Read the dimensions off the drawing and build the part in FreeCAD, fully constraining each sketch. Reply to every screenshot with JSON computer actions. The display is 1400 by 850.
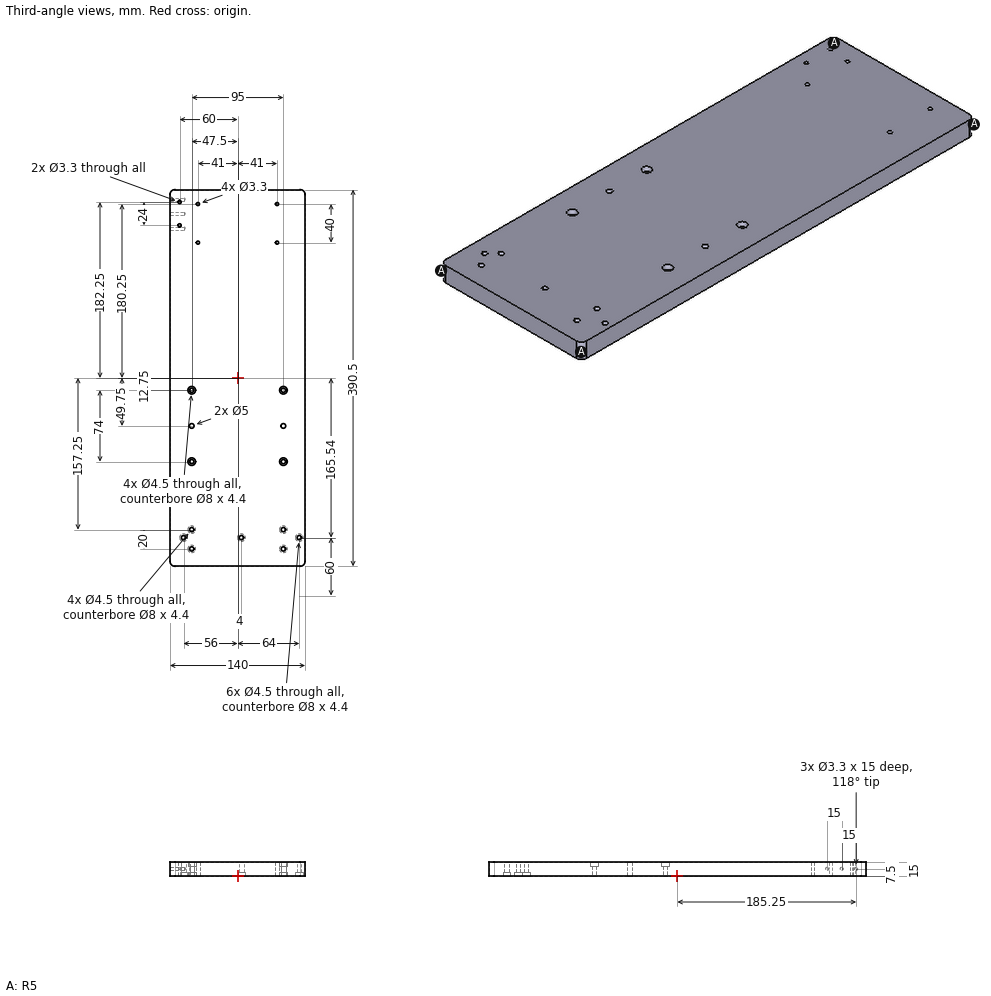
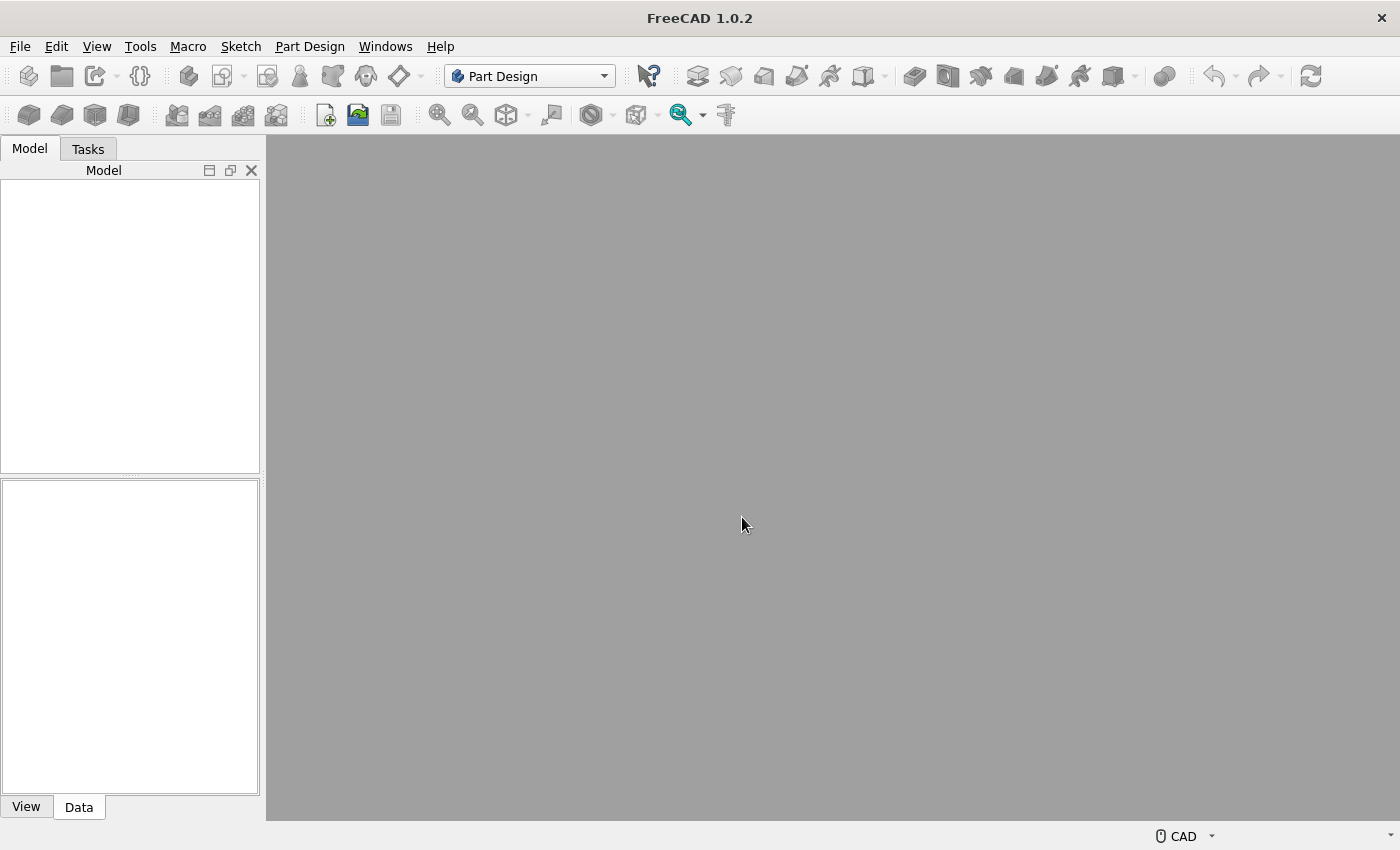
{"action": "left_click", "coordinate": [325, 116]}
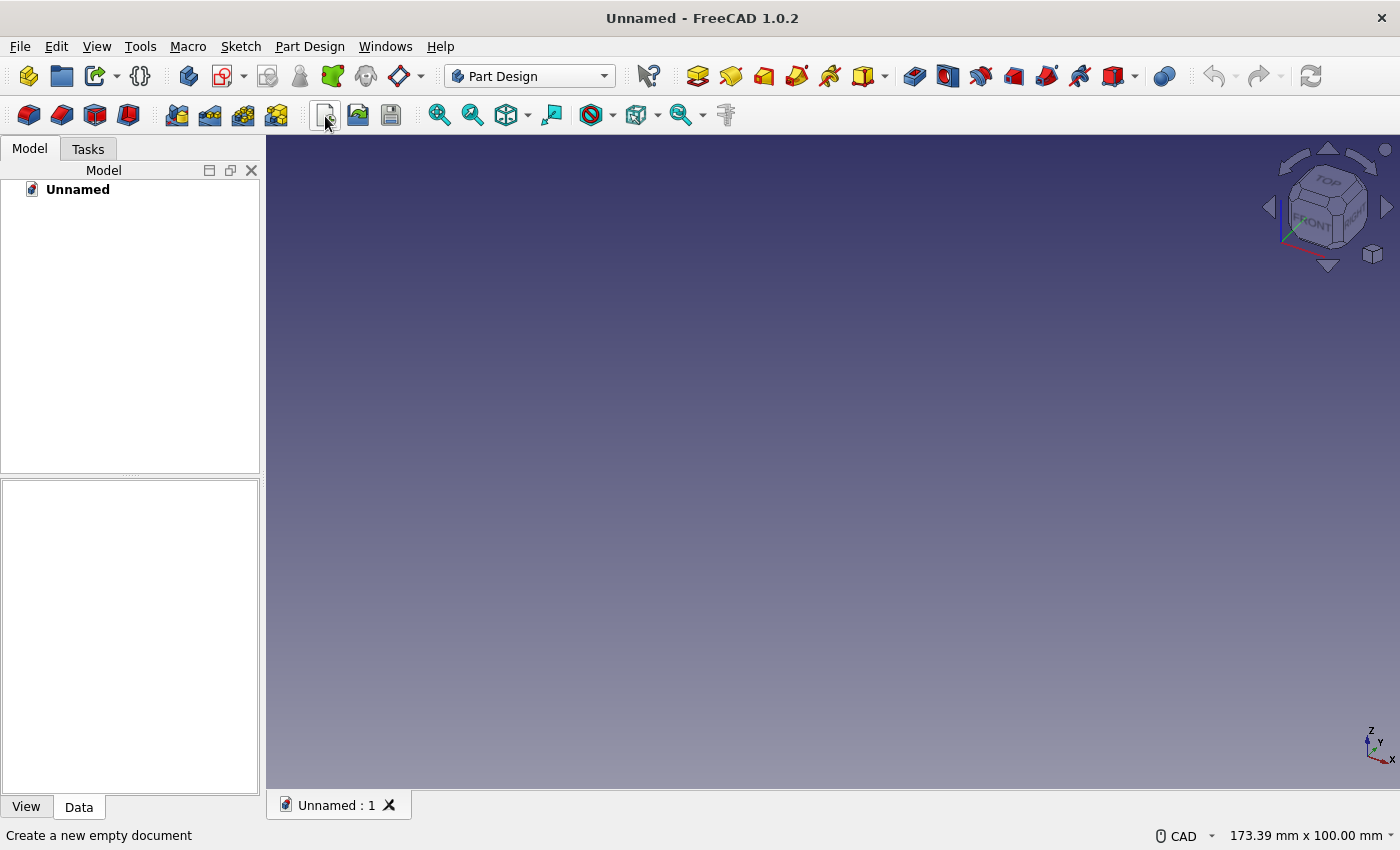
{"action": "left_click", "coordinate": [222, 76]}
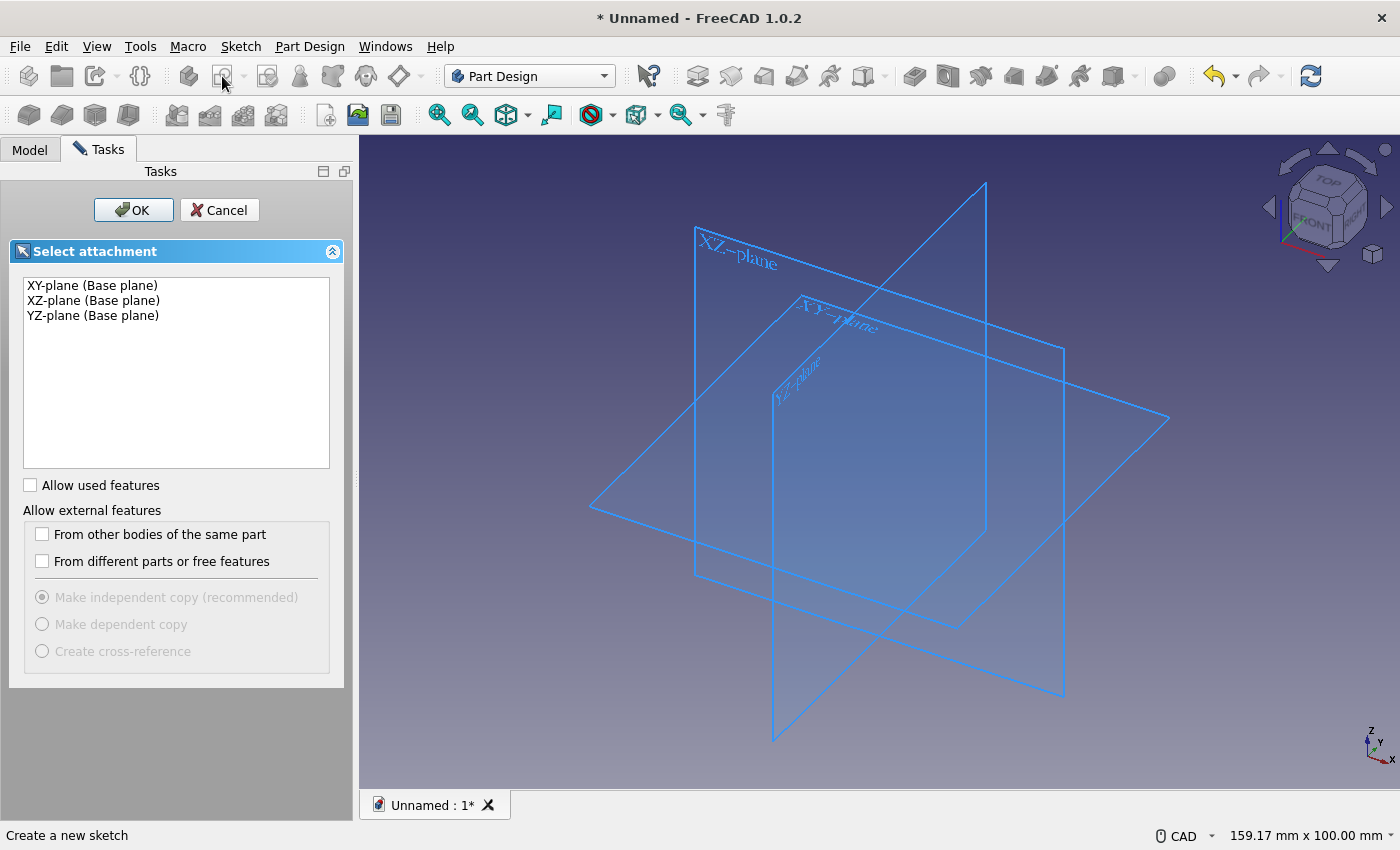
{"action": "left_click", "coordinate": [84, 286]}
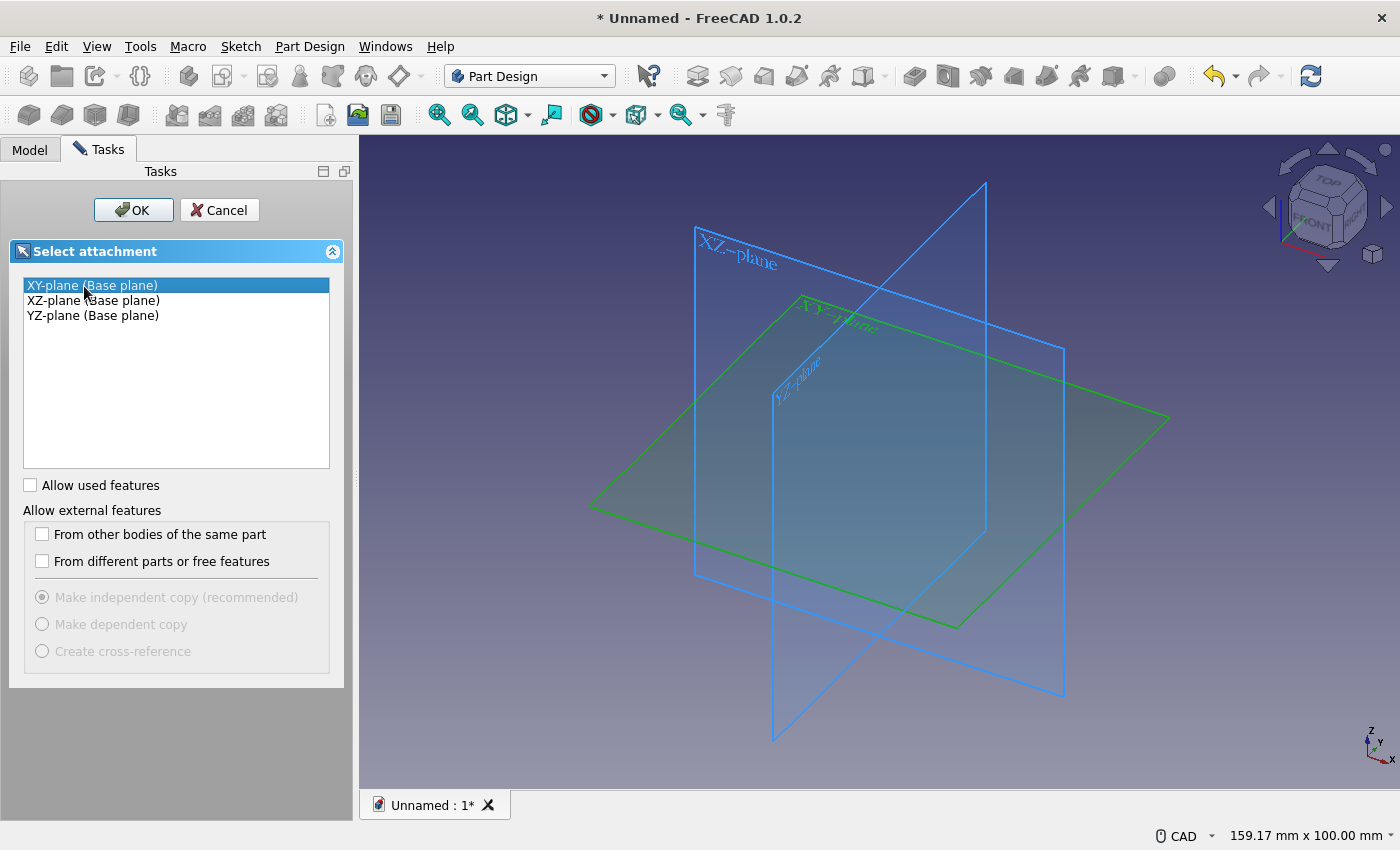
{"action": "left_click", "coordinate": [134, 210]}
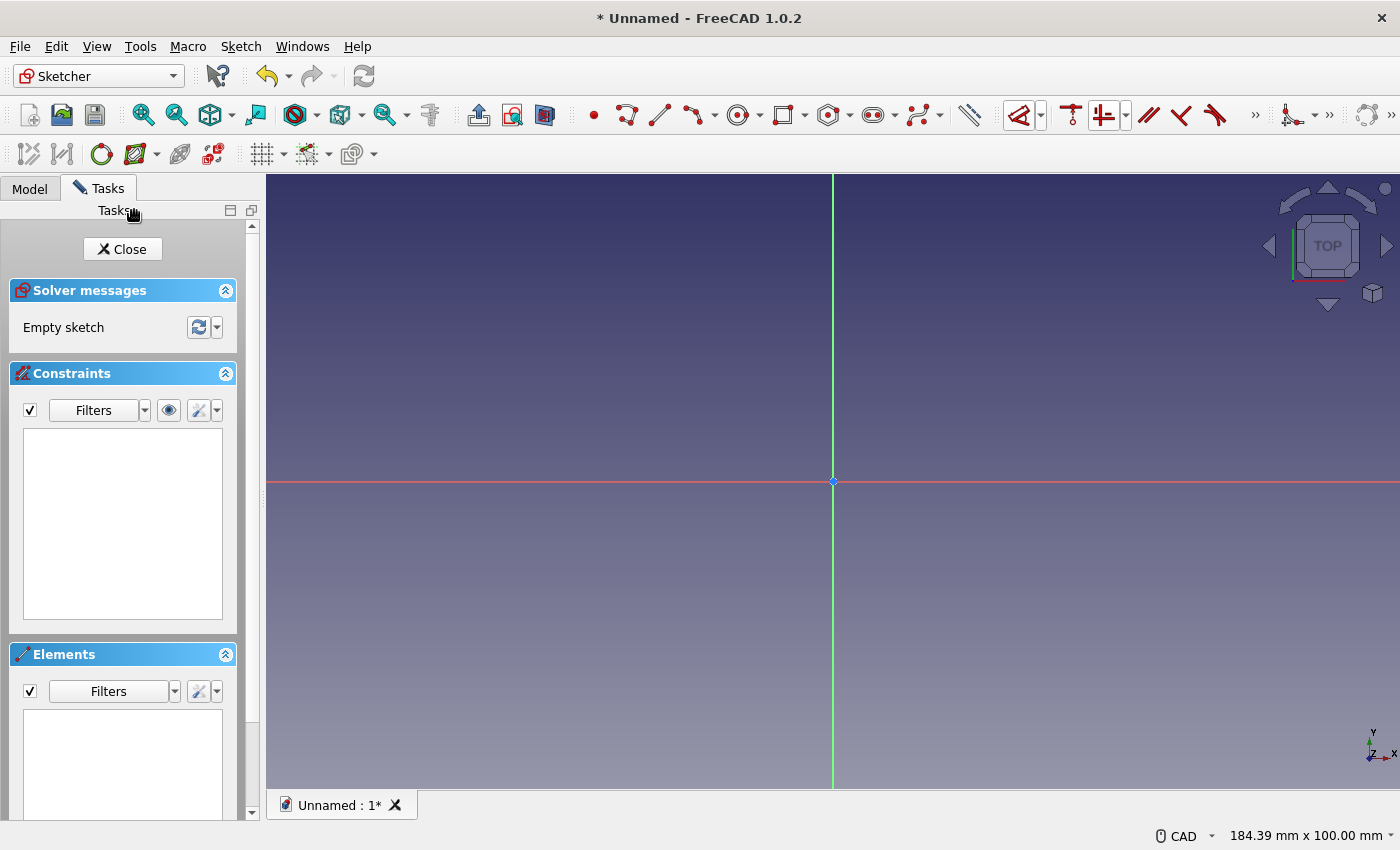
{"action": "scroll", "coordinate": [751, 482], "scroll_direction": "down", "scroll_amount": 9}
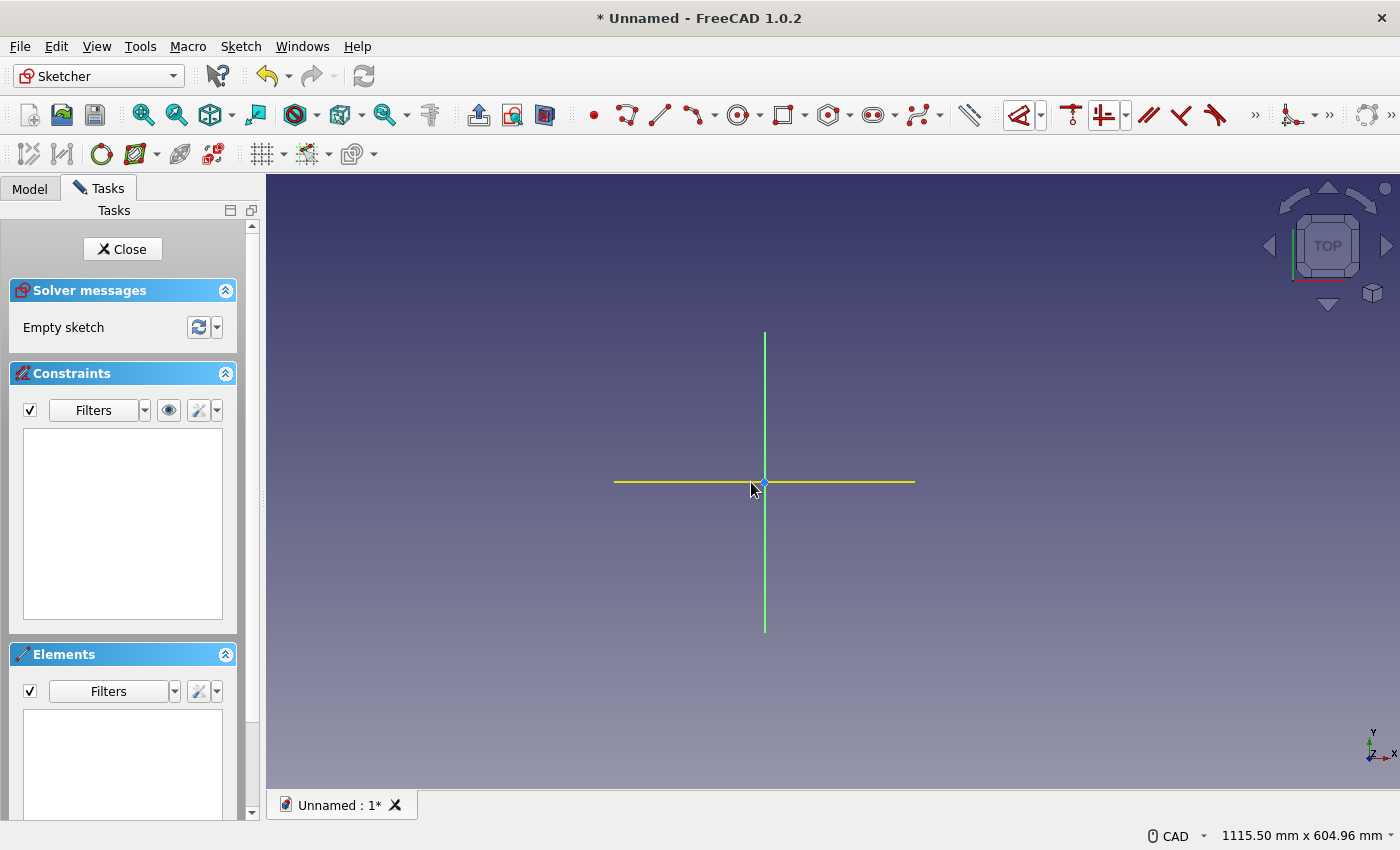
{"action": "left_click", "coordinate": [804, 116]}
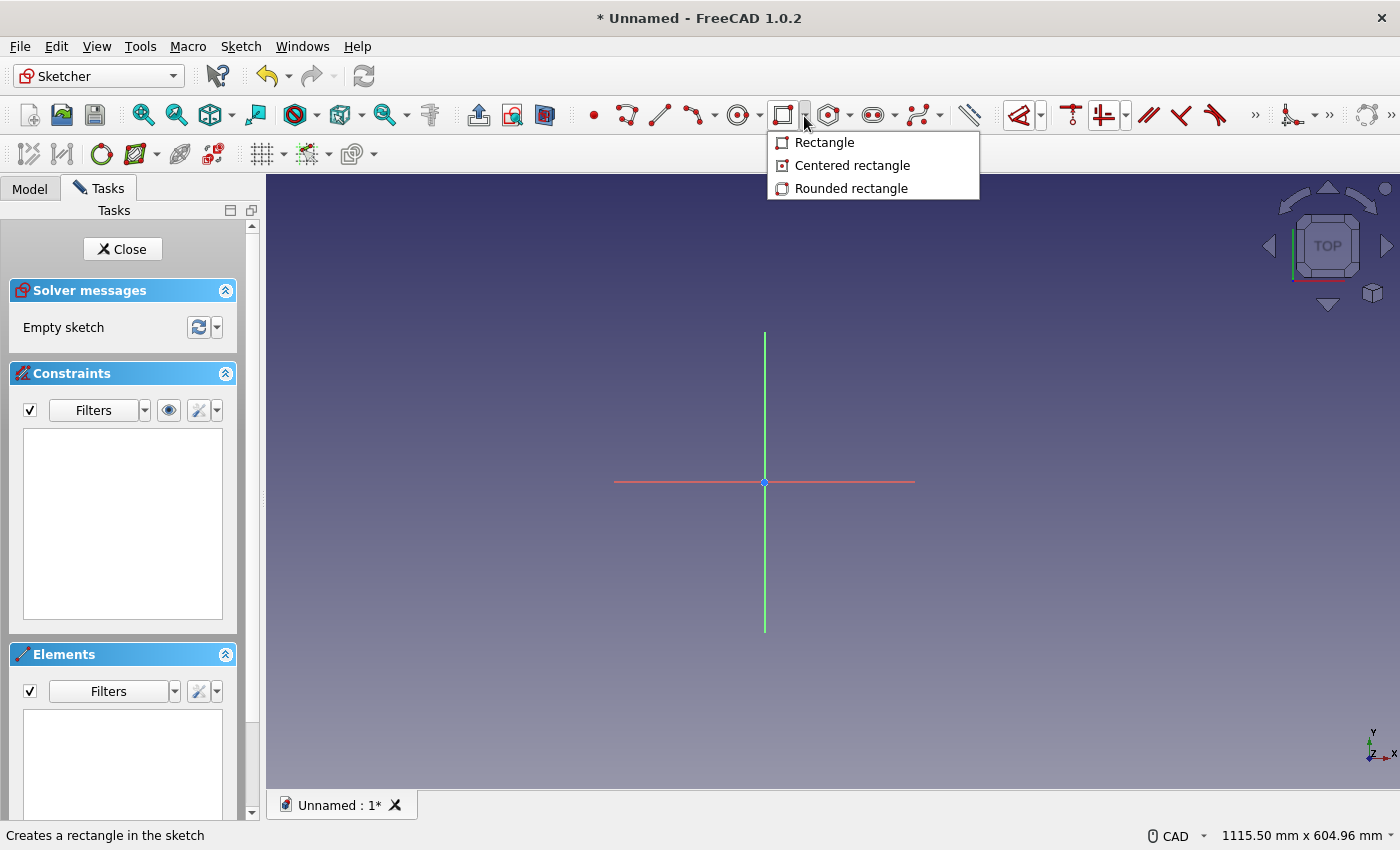
{"action": "left_click", "coordinate": [874, 166]}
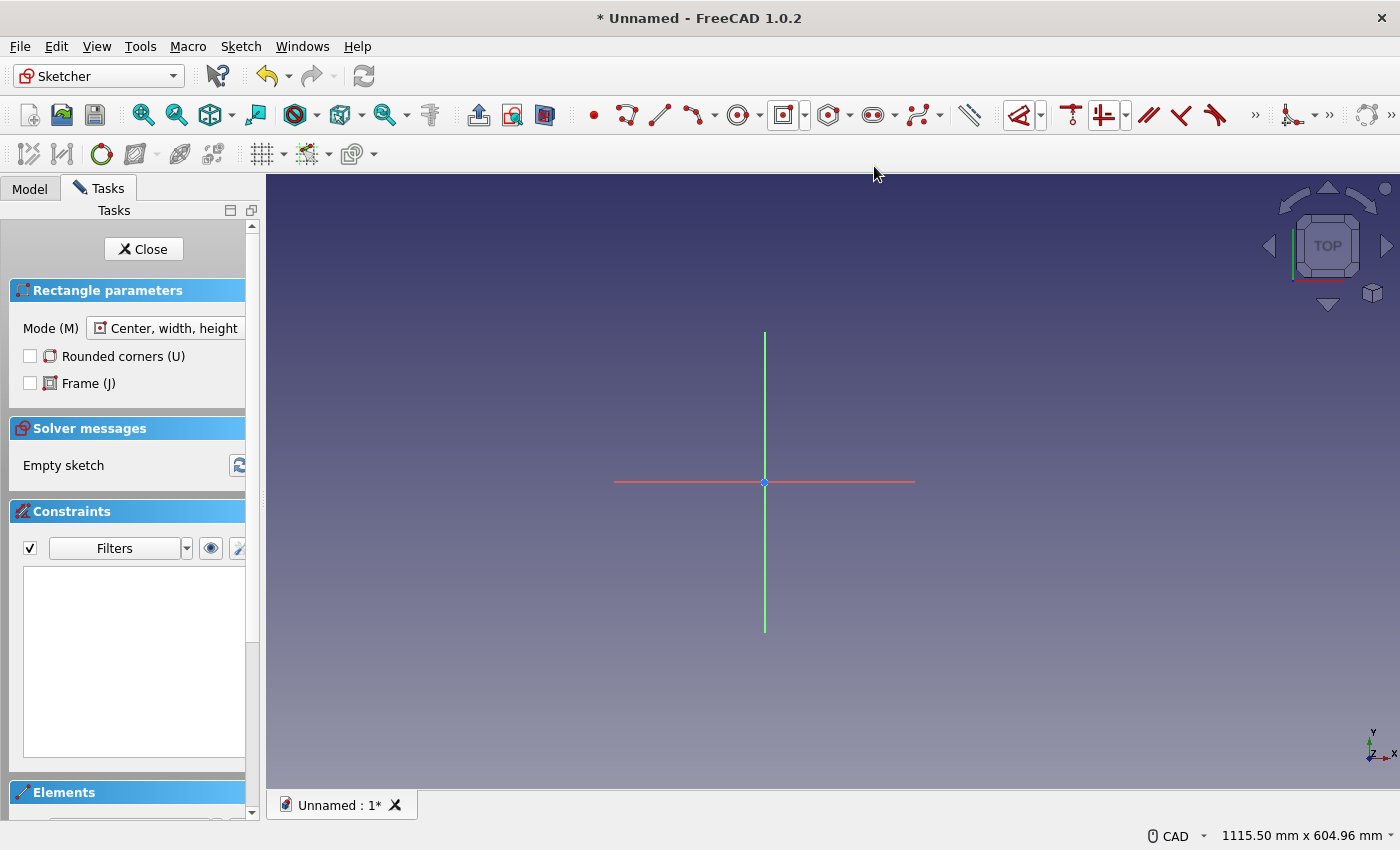
{"action": "left_click", "coordinate": [765, 482]}
{"action": "mouse_move", "coordinate": [836, 284]}